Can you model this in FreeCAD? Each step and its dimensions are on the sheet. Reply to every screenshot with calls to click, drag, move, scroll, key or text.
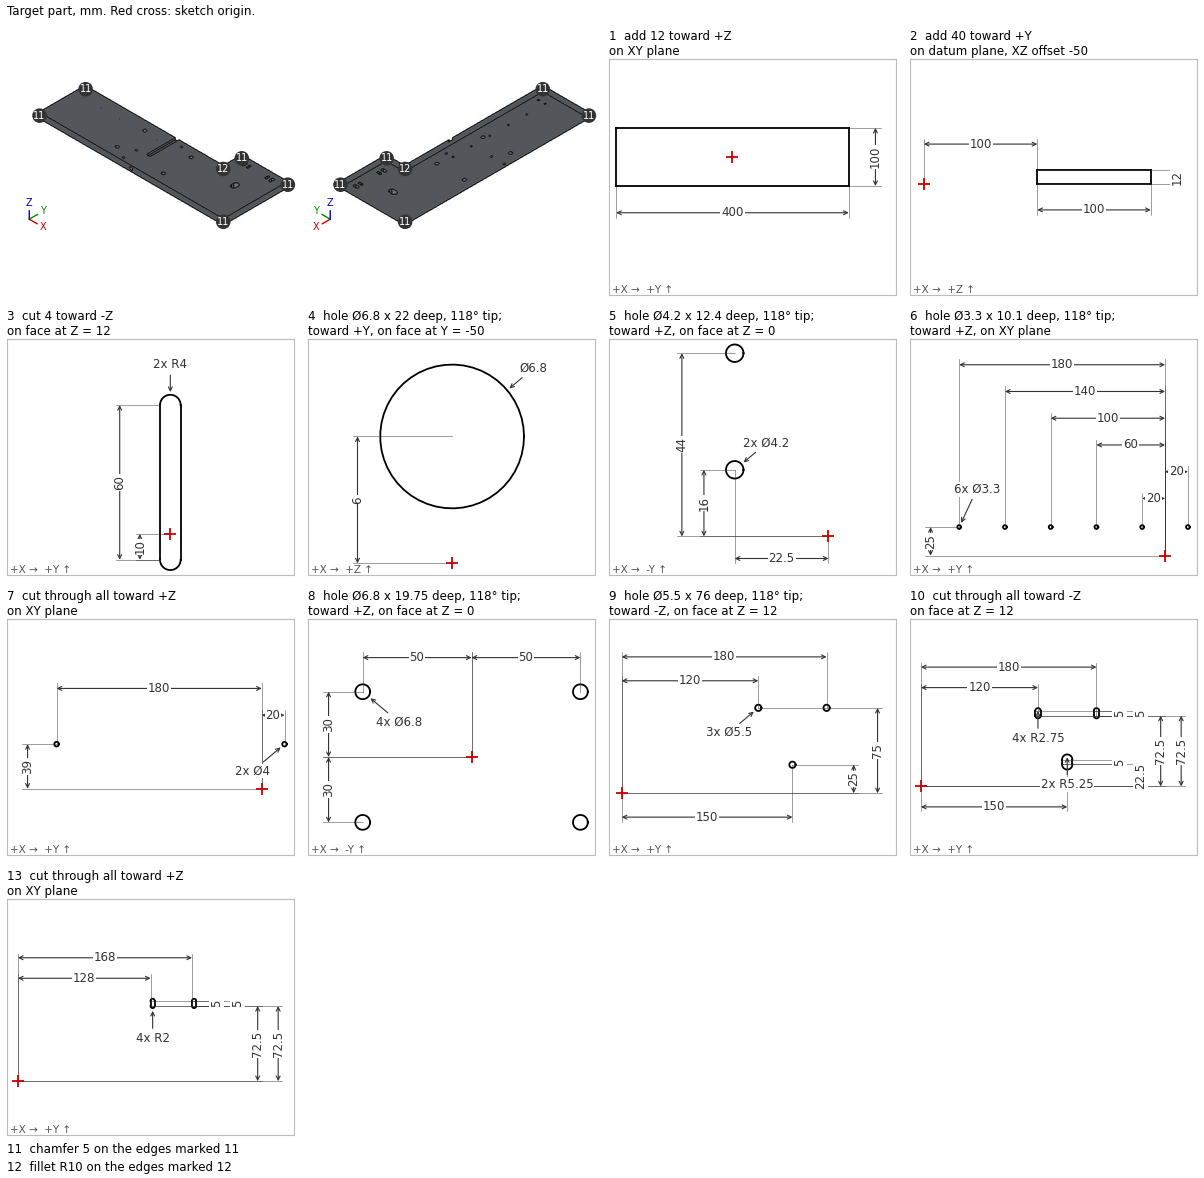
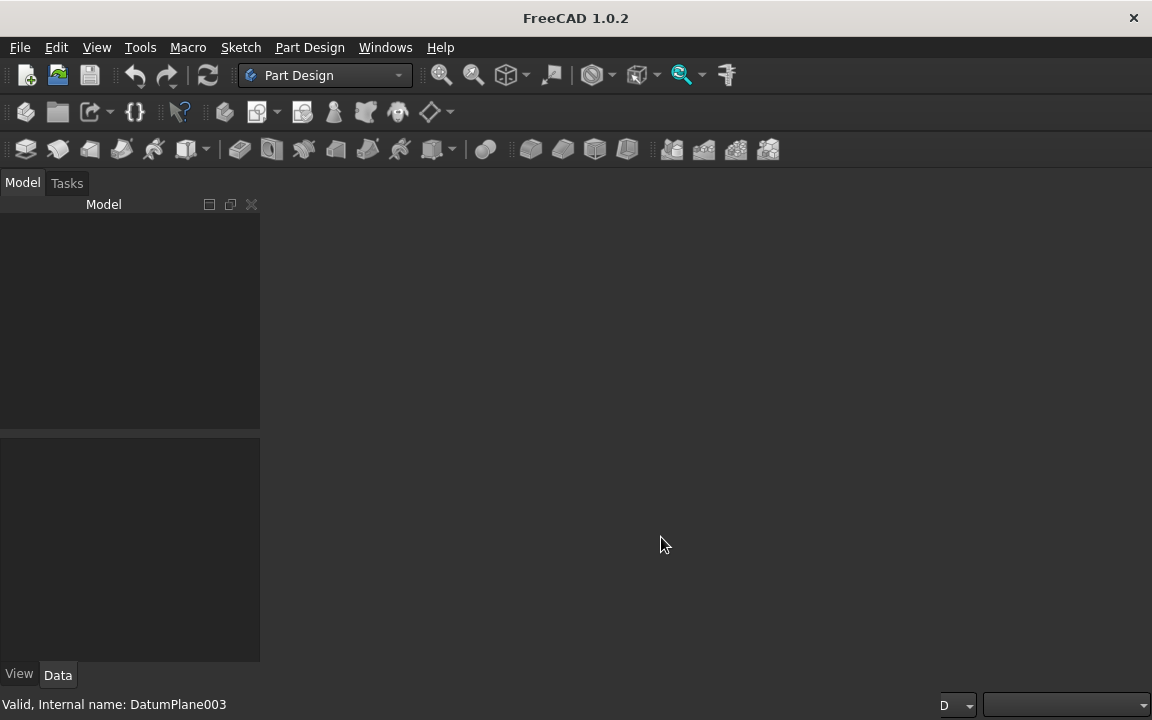
click(26, 76)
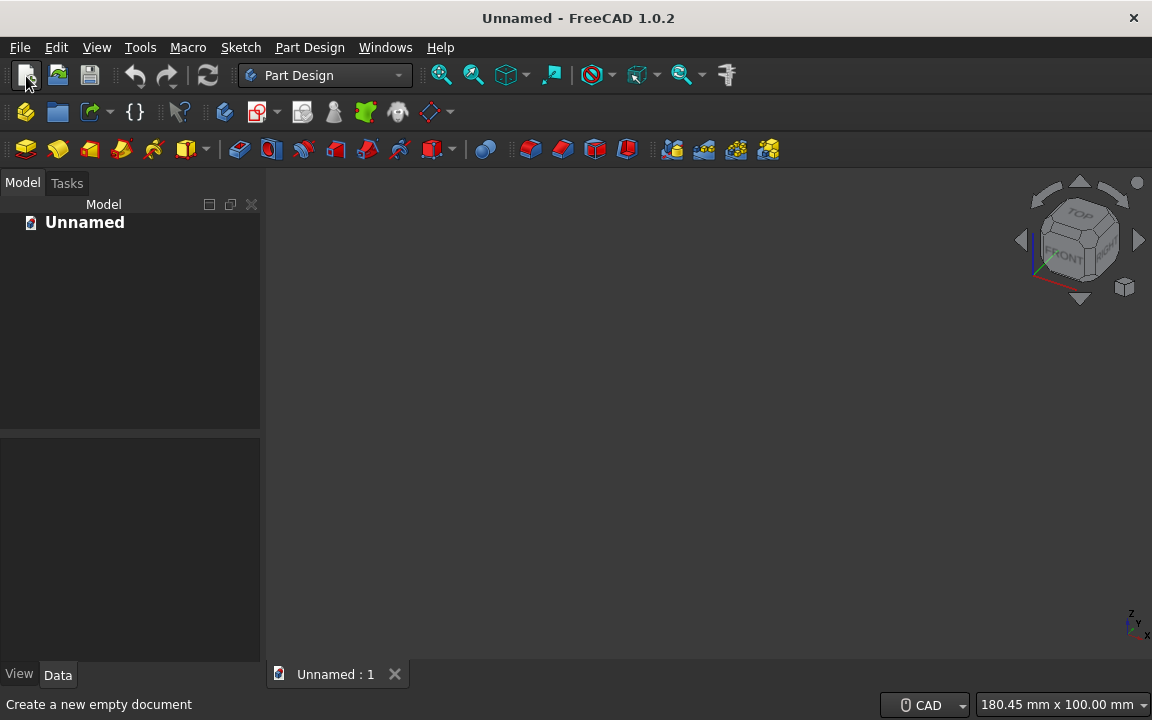
click(258, 112)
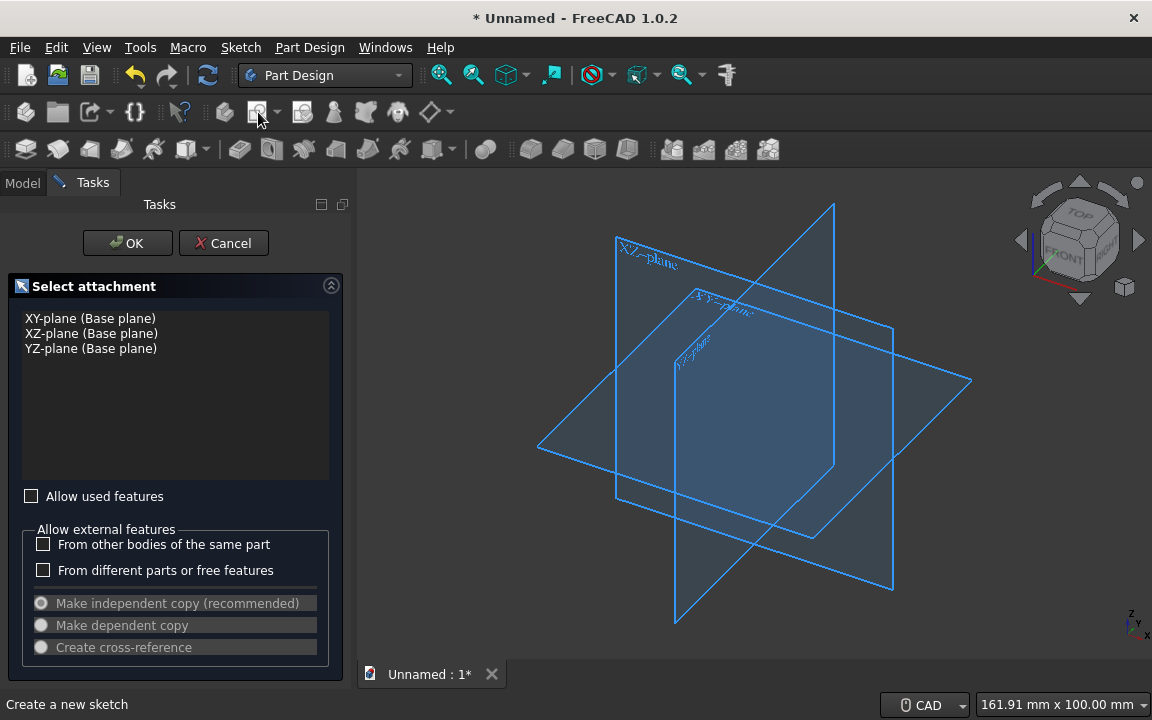
click(82, 318)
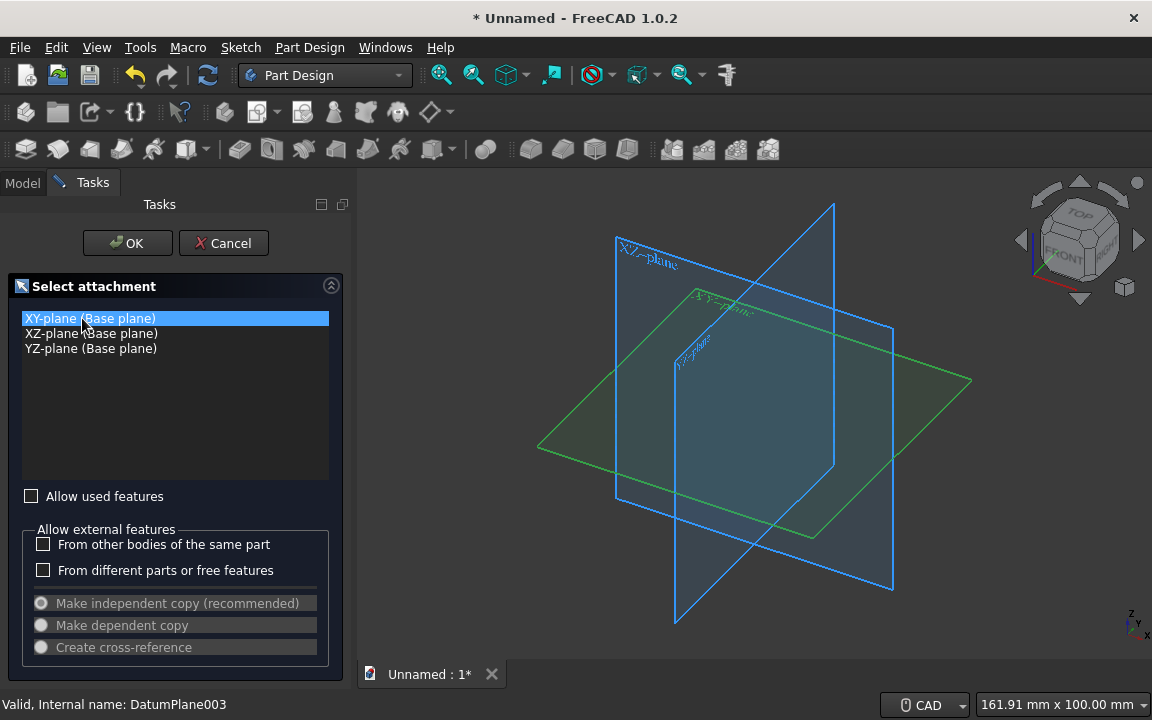
click(128, 243)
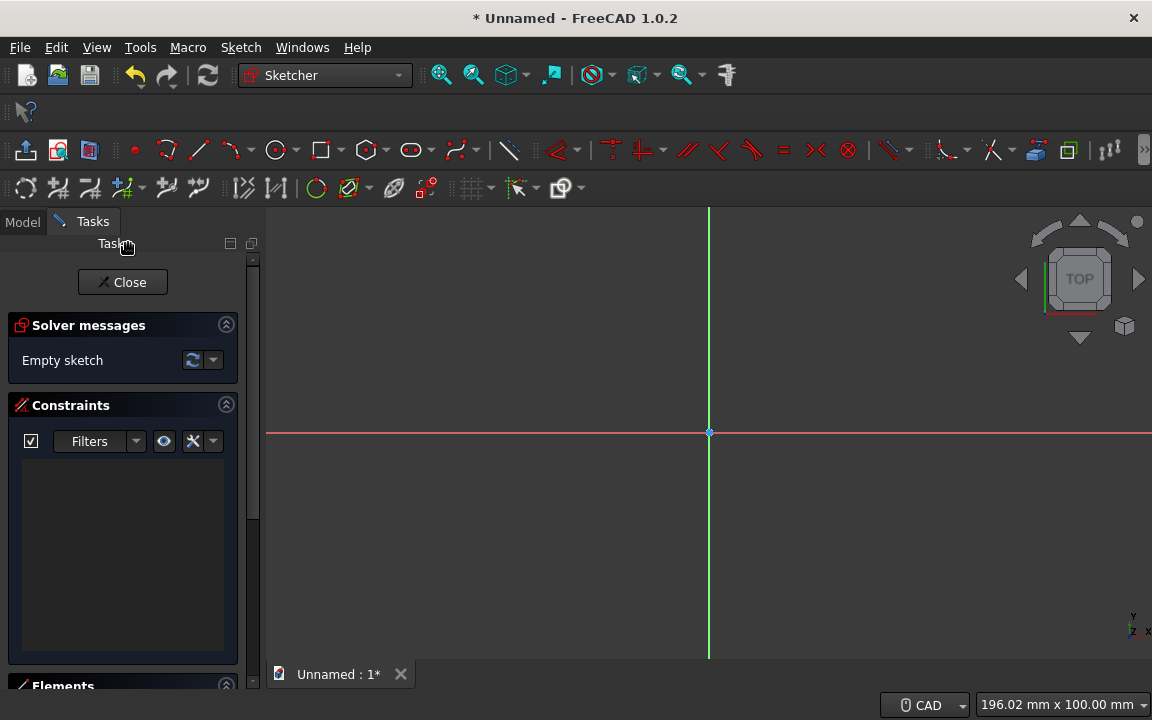
scroll(618, 433, down, 7)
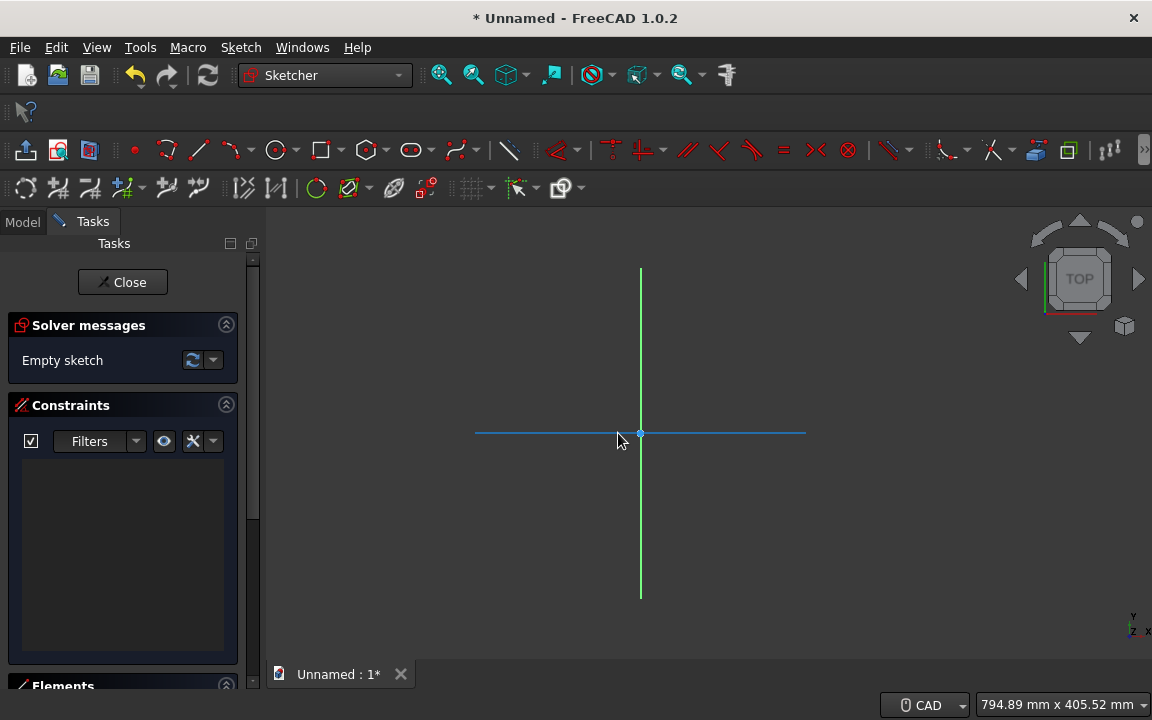
key(g)
key(v)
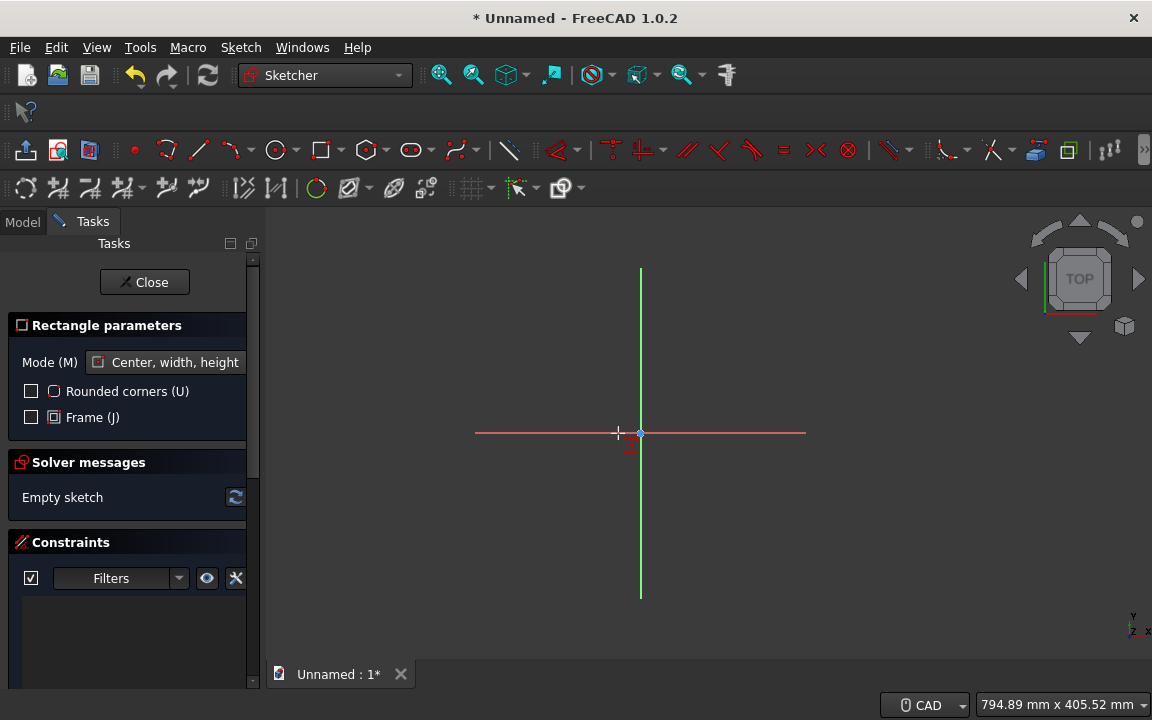
click(641, 433)
move(864, 378)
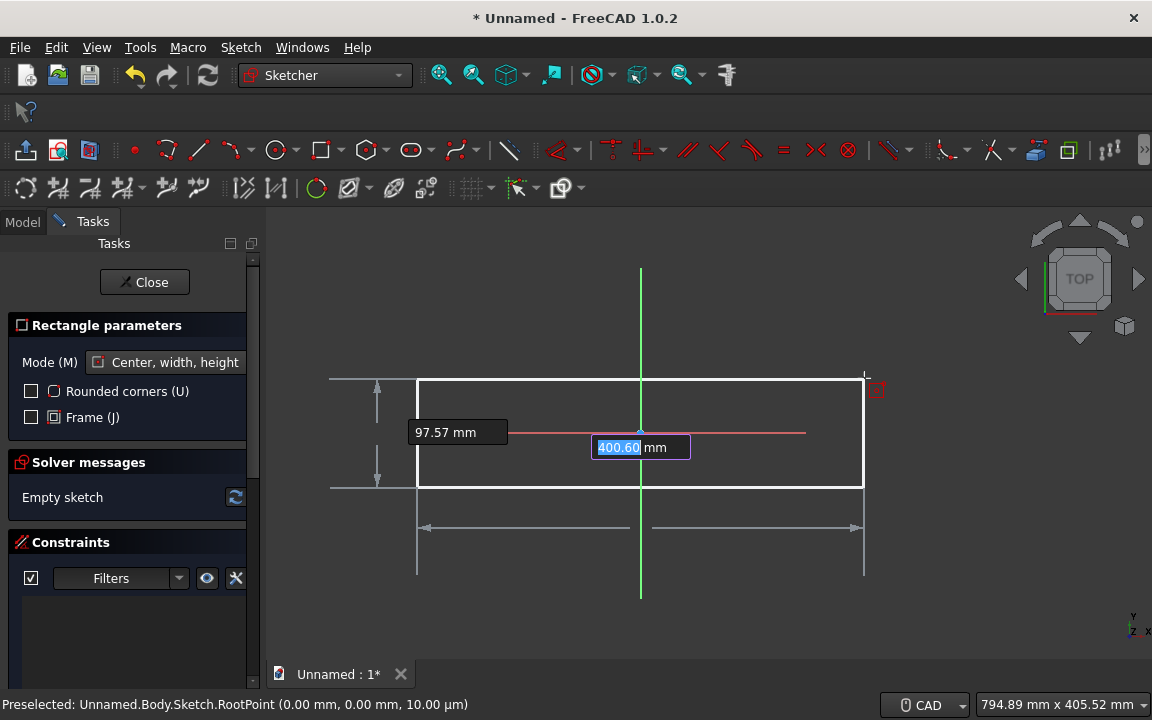
text(400)
key(Tab)
text(100)
key(Return)
key(Escape)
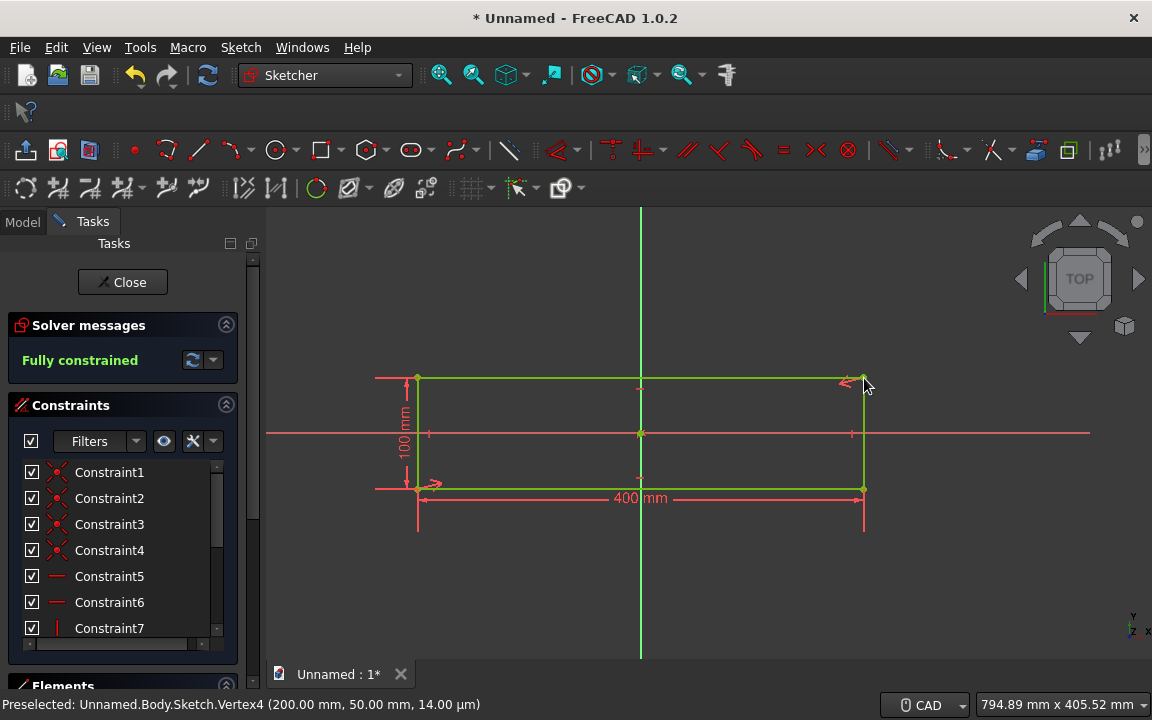
click(123, 282)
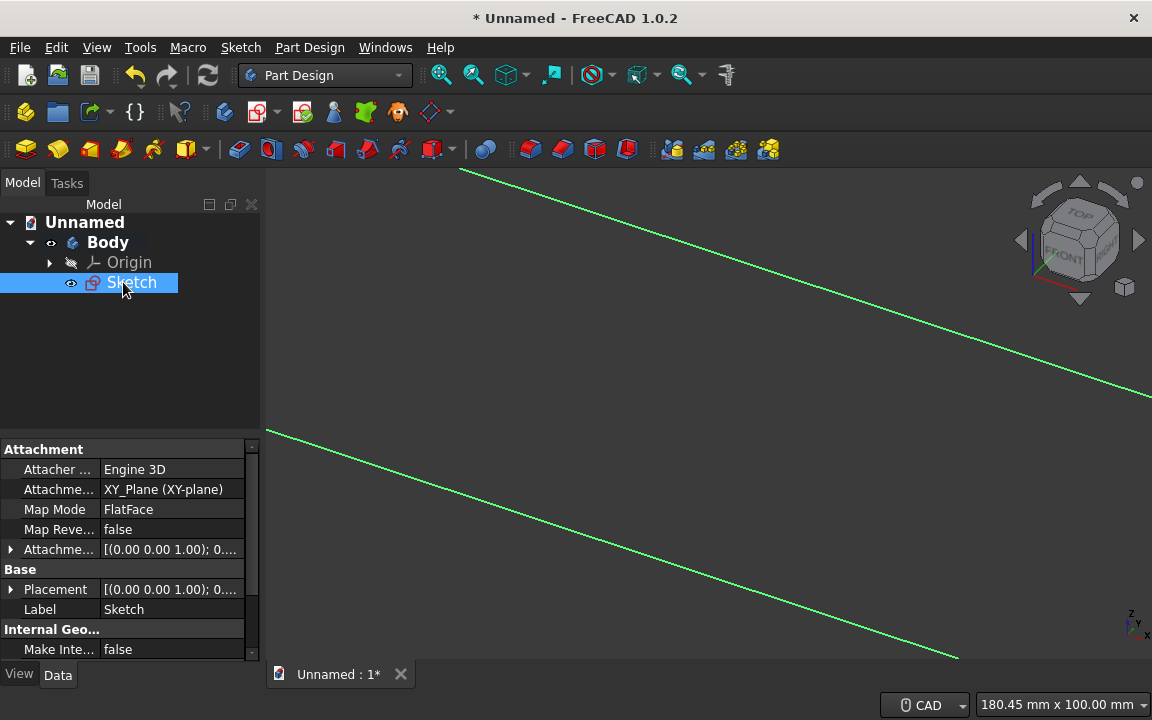
click(26, 150)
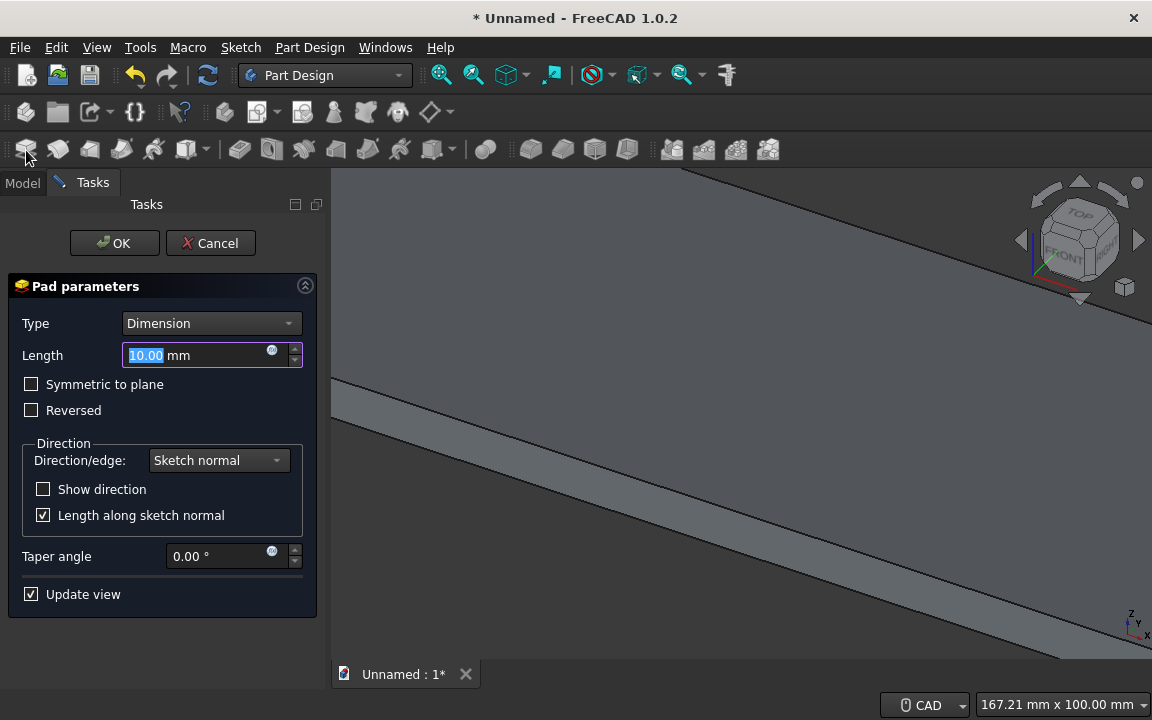
text(12)
key(Tab)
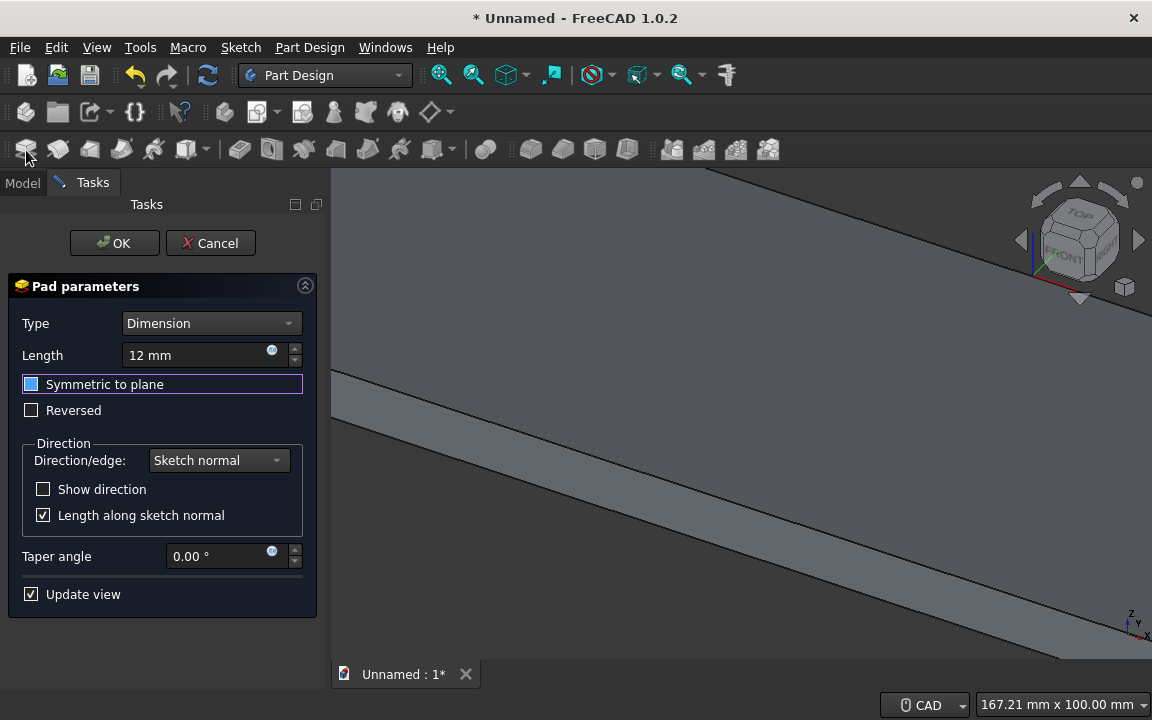
click(115, 243)